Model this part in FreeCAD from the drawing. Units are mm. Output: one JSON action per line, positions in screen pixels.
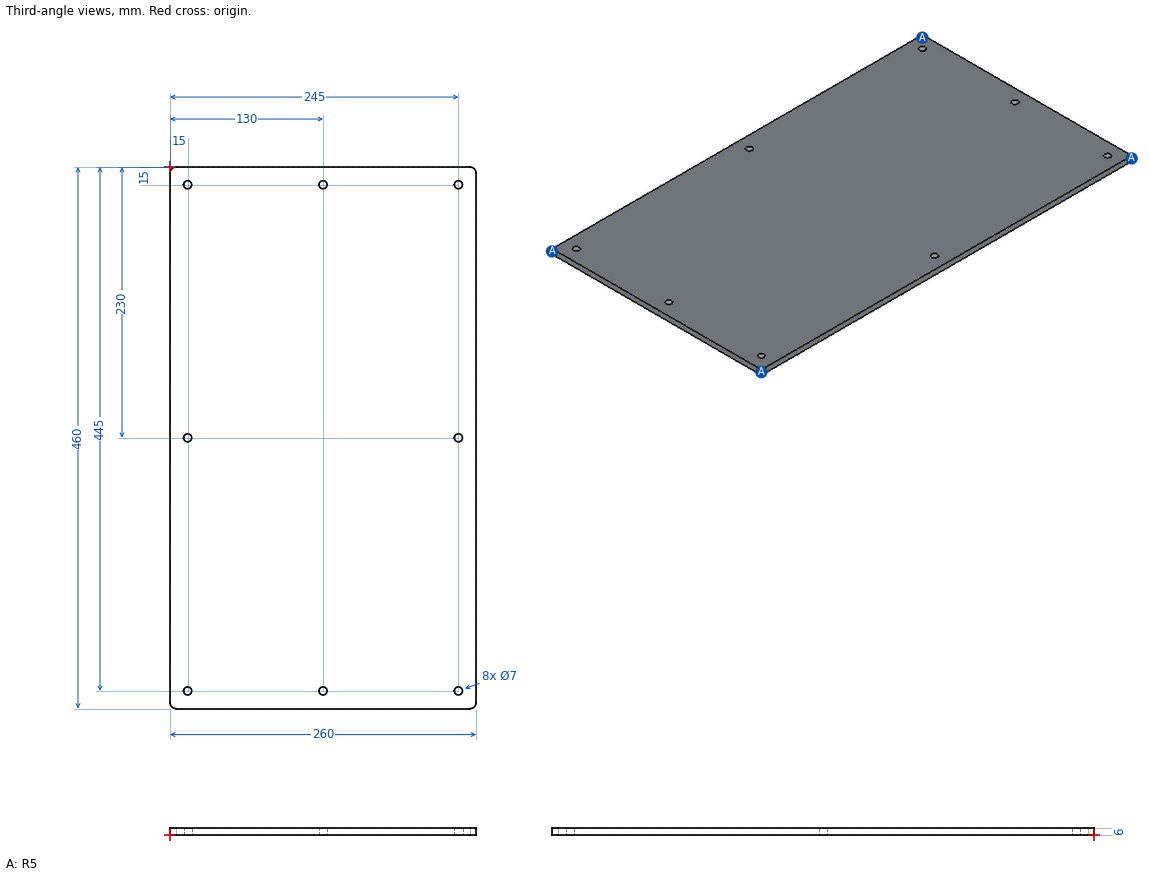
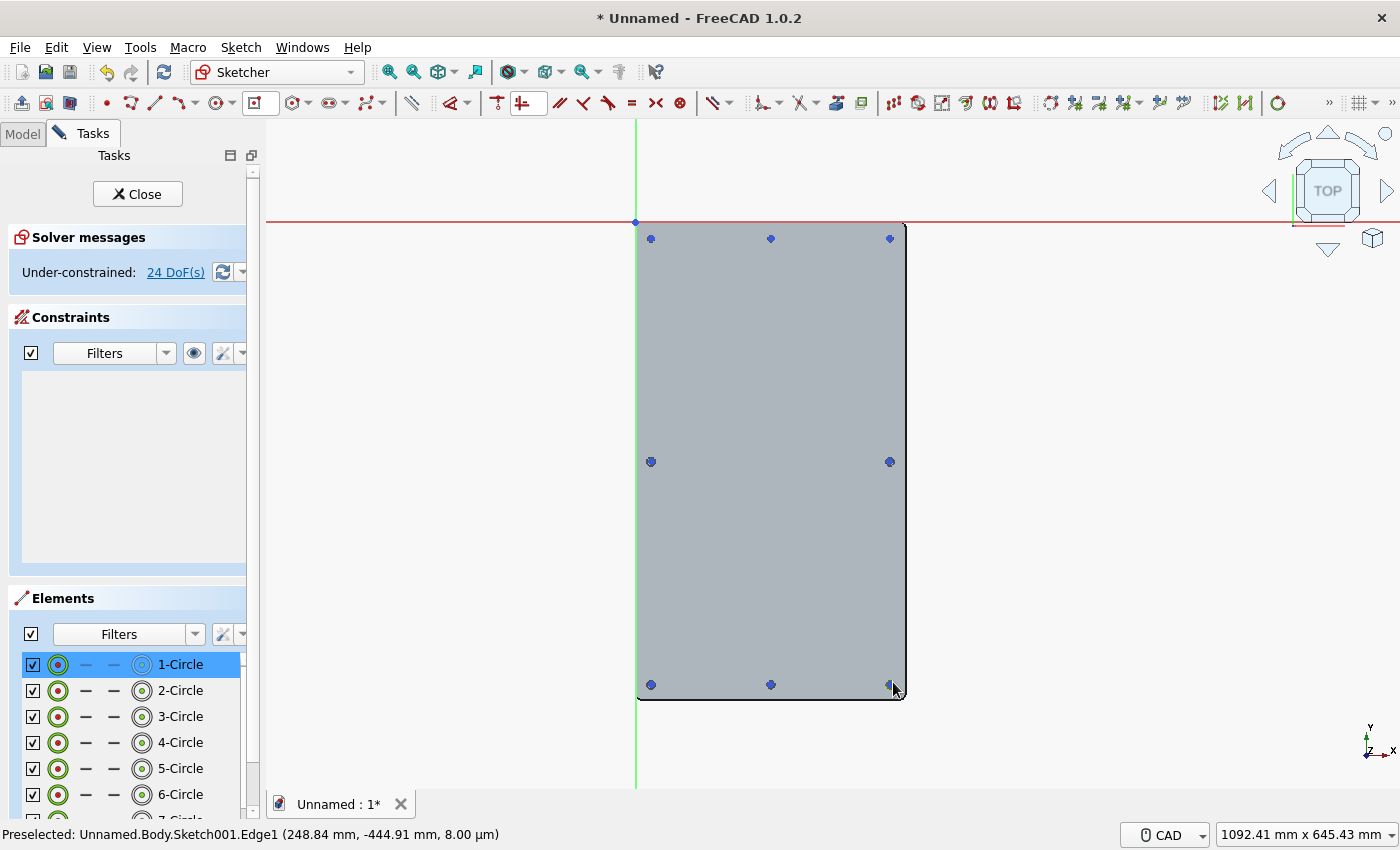
{"action": "scroll", "coordinate": [654, 682], "scroll_direction": "up", "scroll_amount": 7}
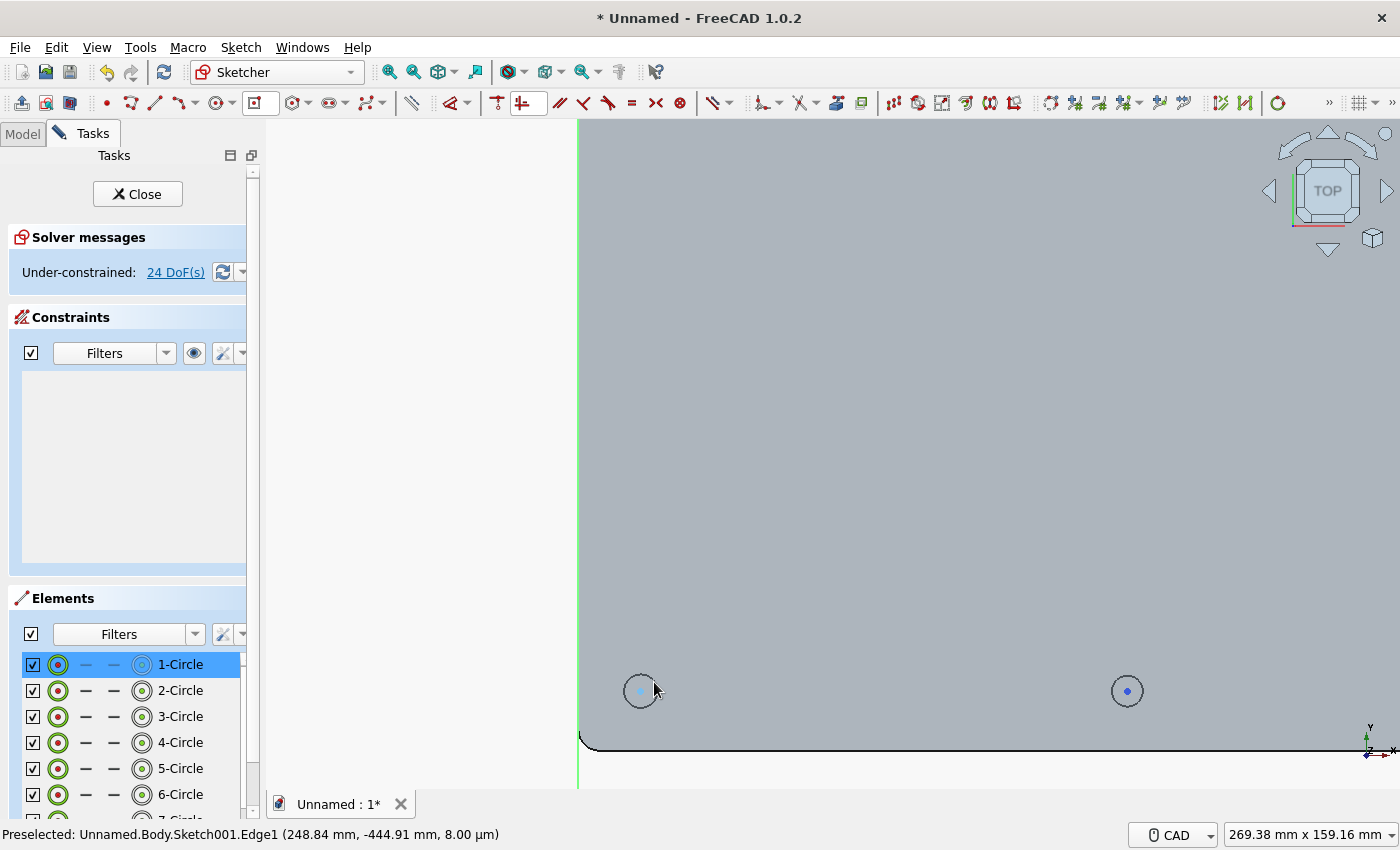
{"action": "left_click", "coordinate": [653, 679]}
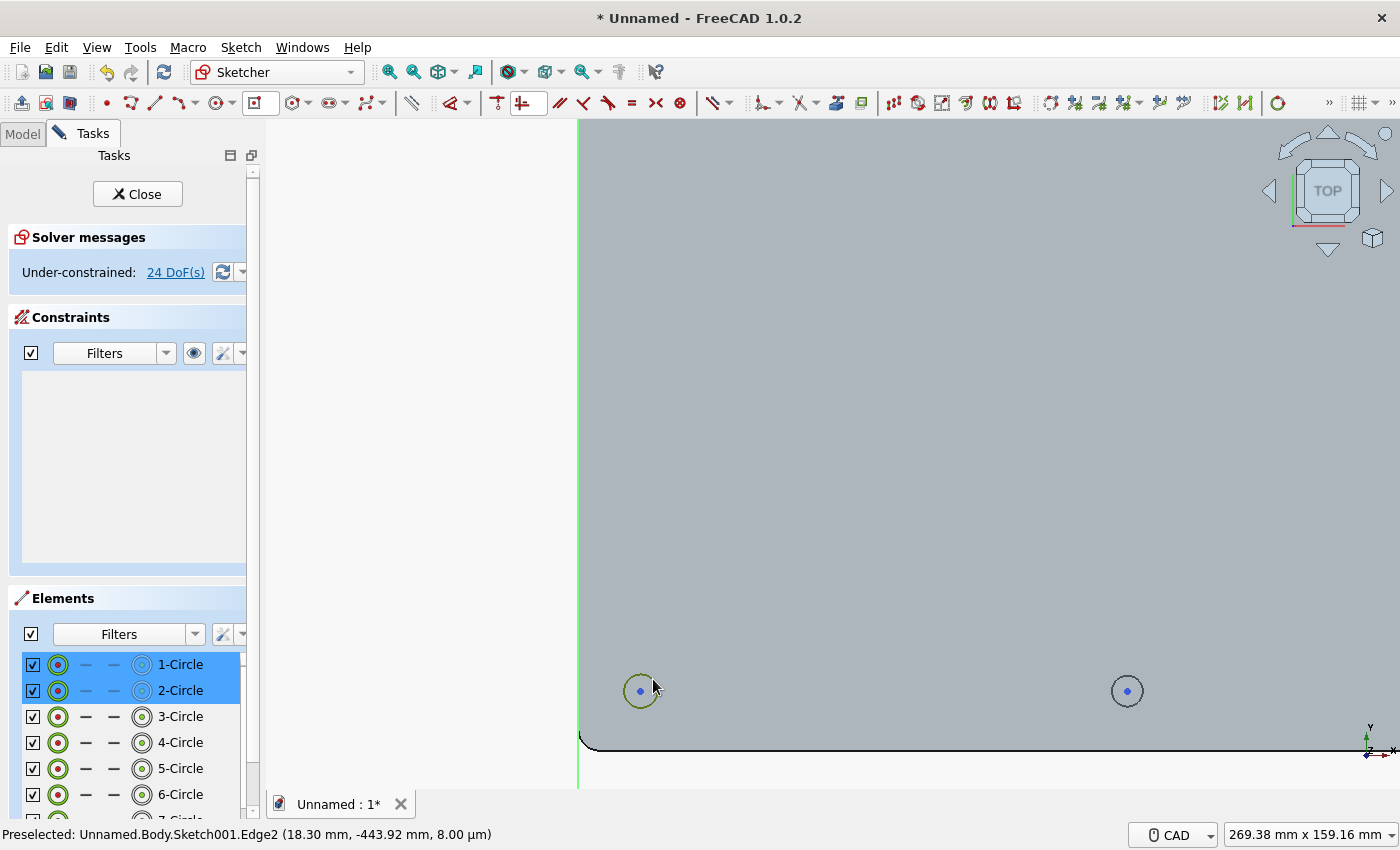
{"action": "scroll", "coordinate": [654, 682], "scroll_direction": "down", "scroll_amount": 7}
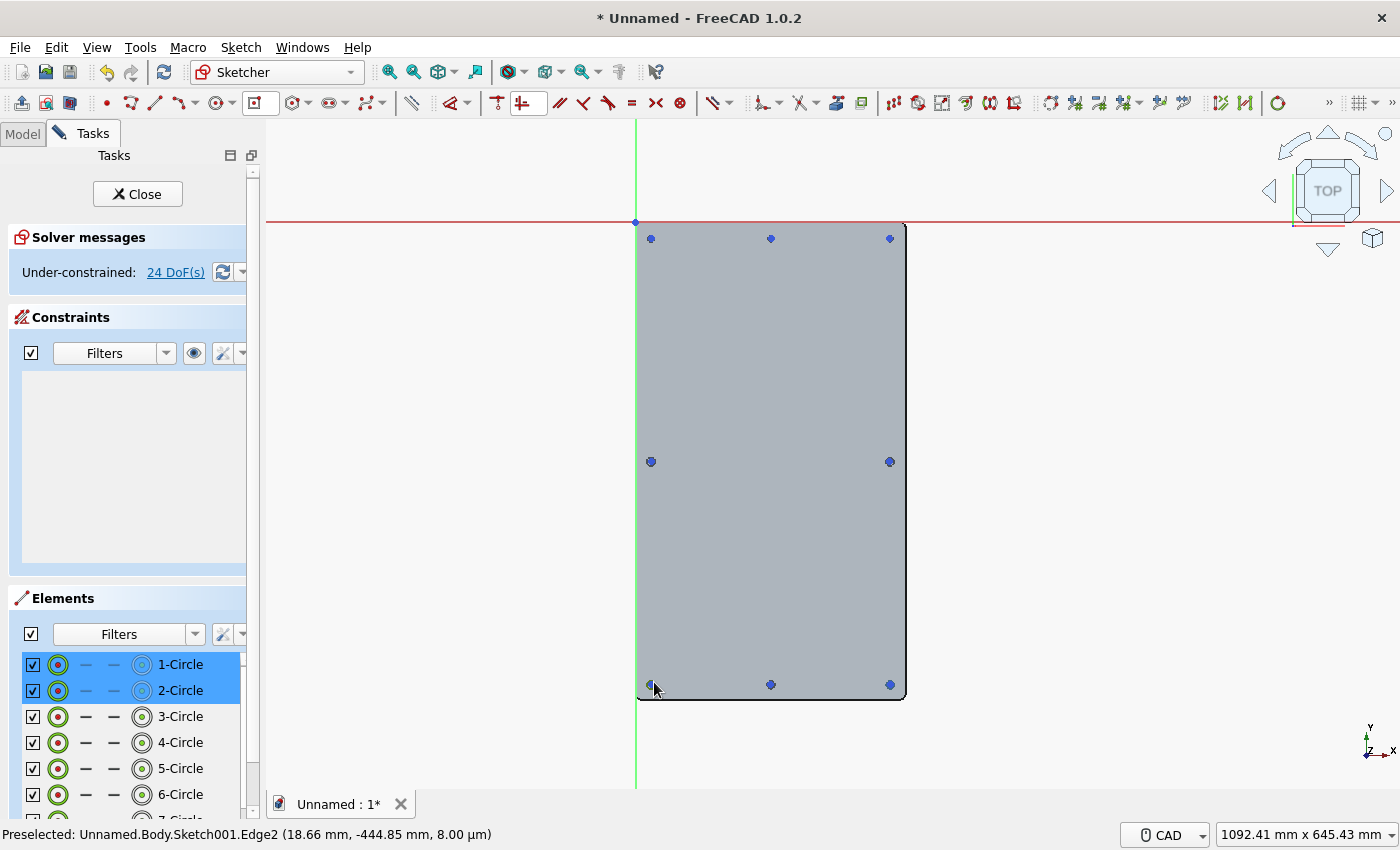
{"action": "scroll", "coordinate": [892, 237], "scroll_direction": "up", "scroll_amount": 8}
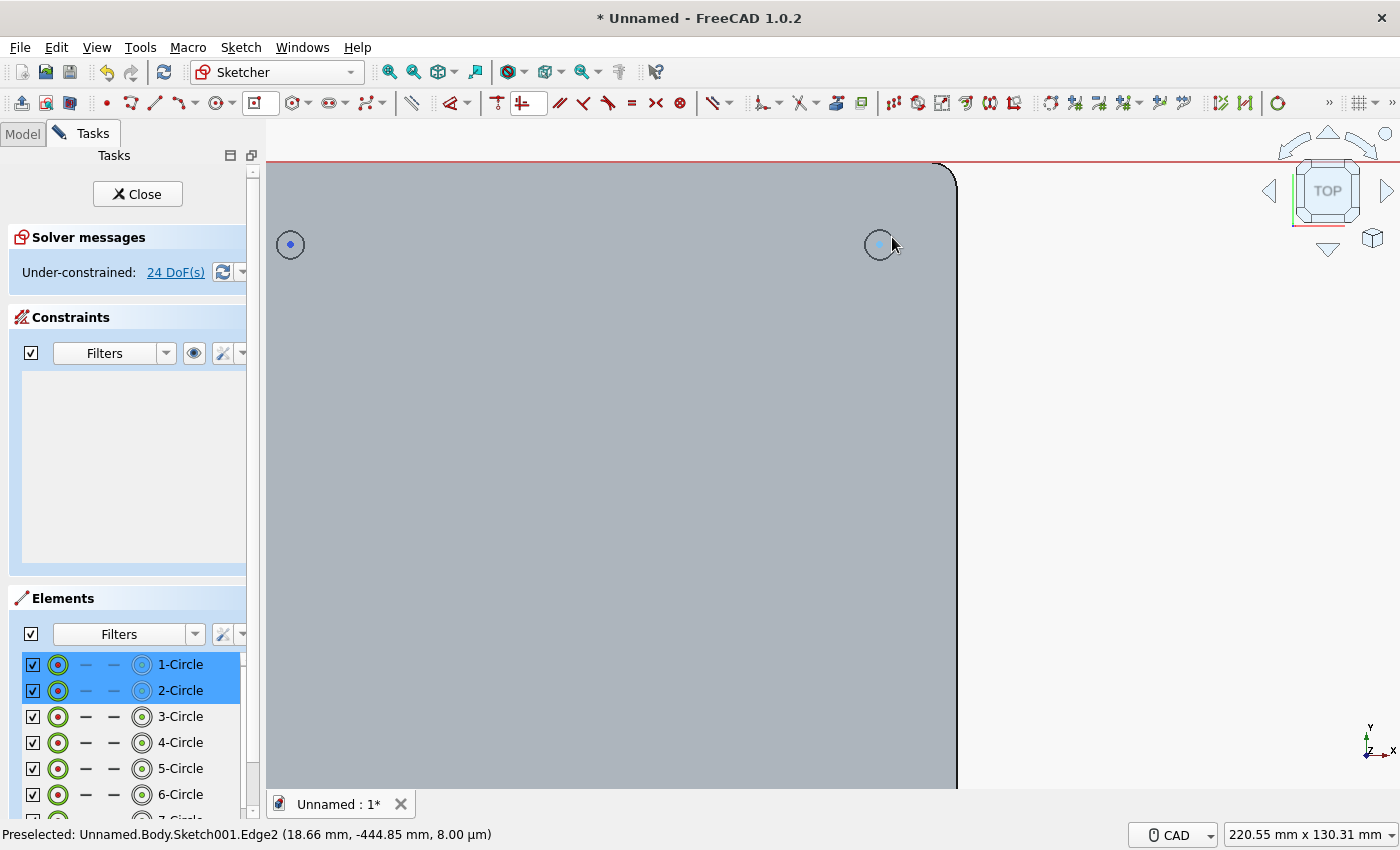
{"action": "left_click", "coordinate": [890, 234]}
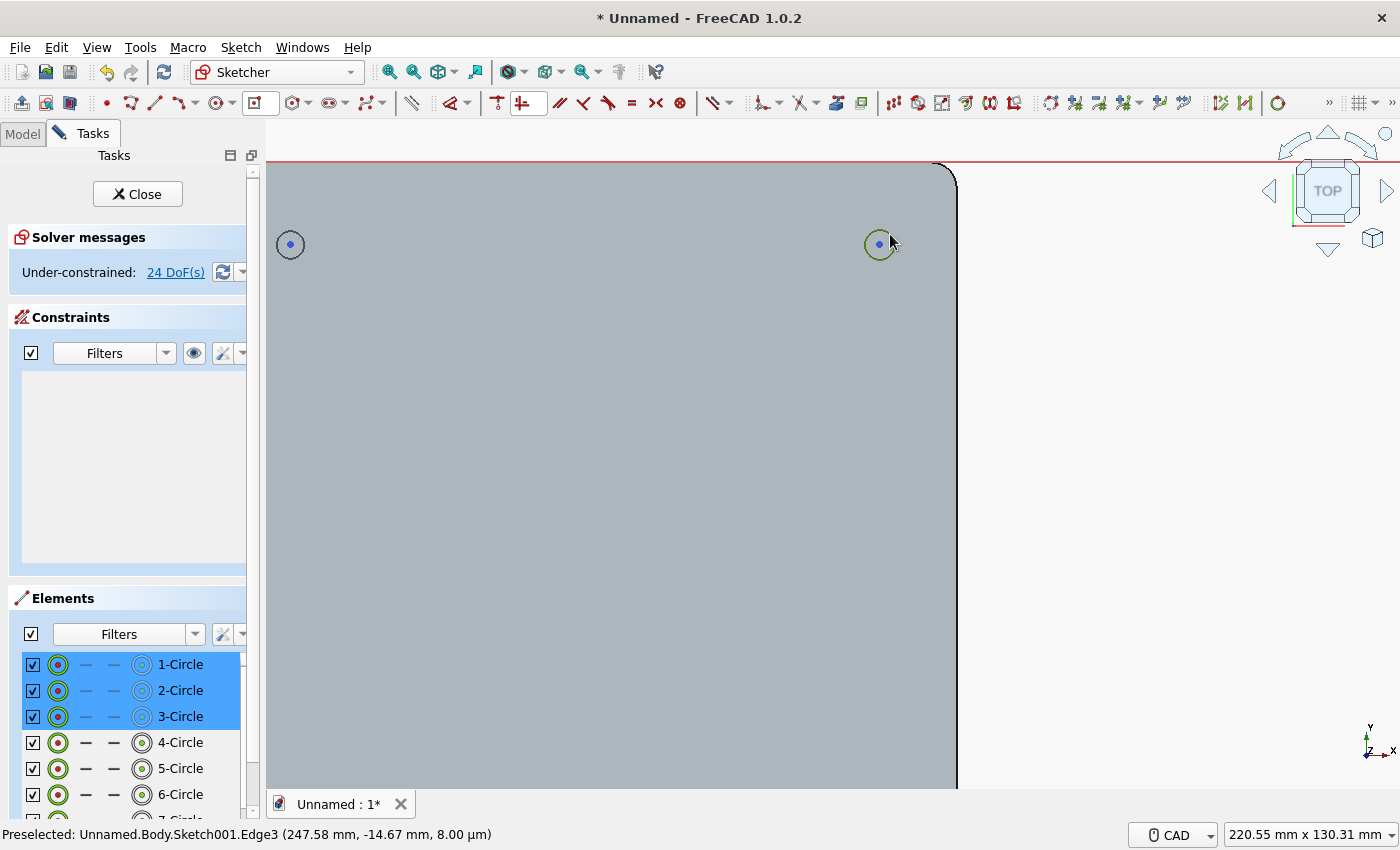
{"action": "scroll", "coordinate": [892, 236], "scroll_direction": "down", "scroll_amount": 8}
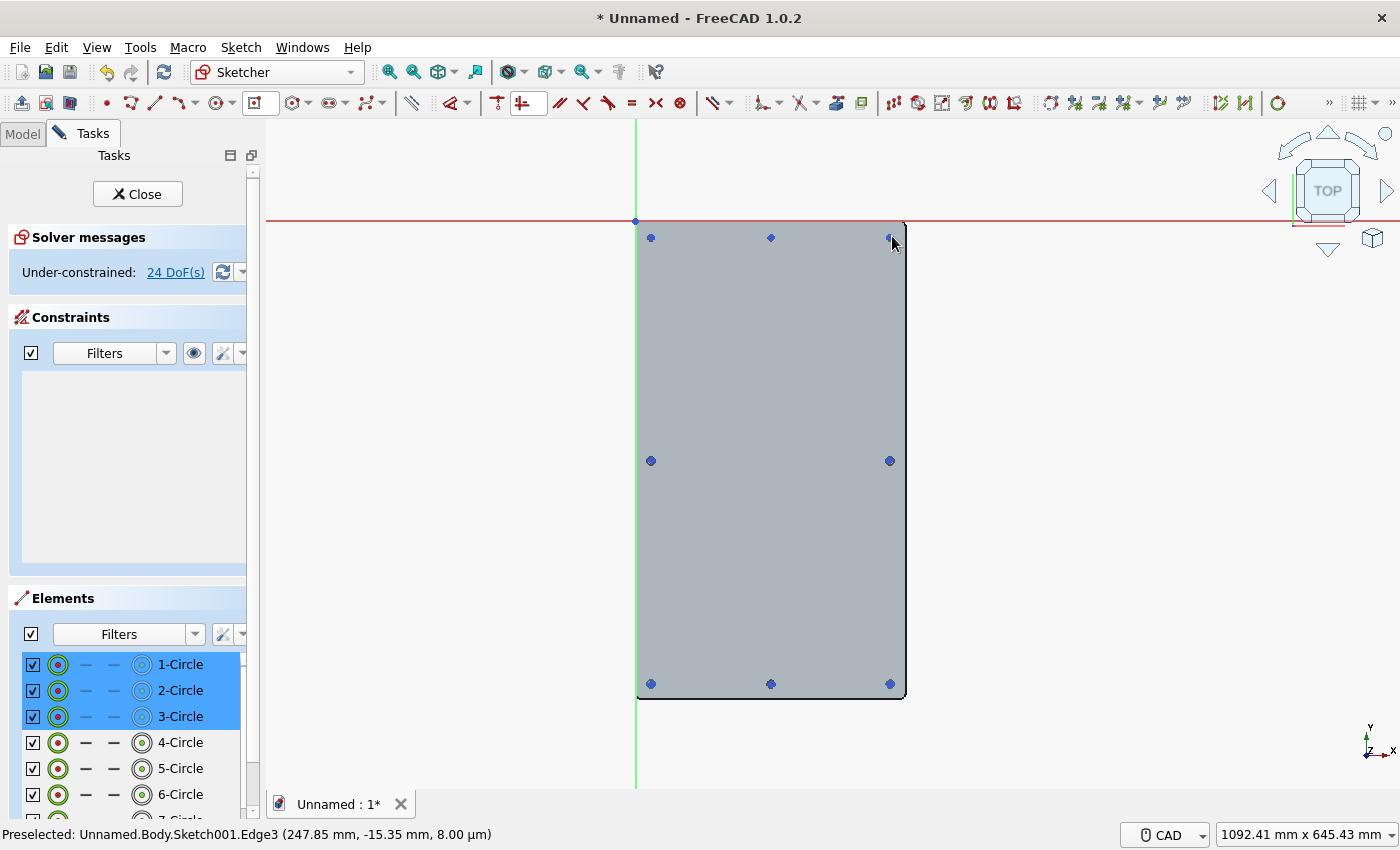
{"action": "scroll", "coordinate": [653, 236], "scroll_direction": "up", "scroll_amount": 8}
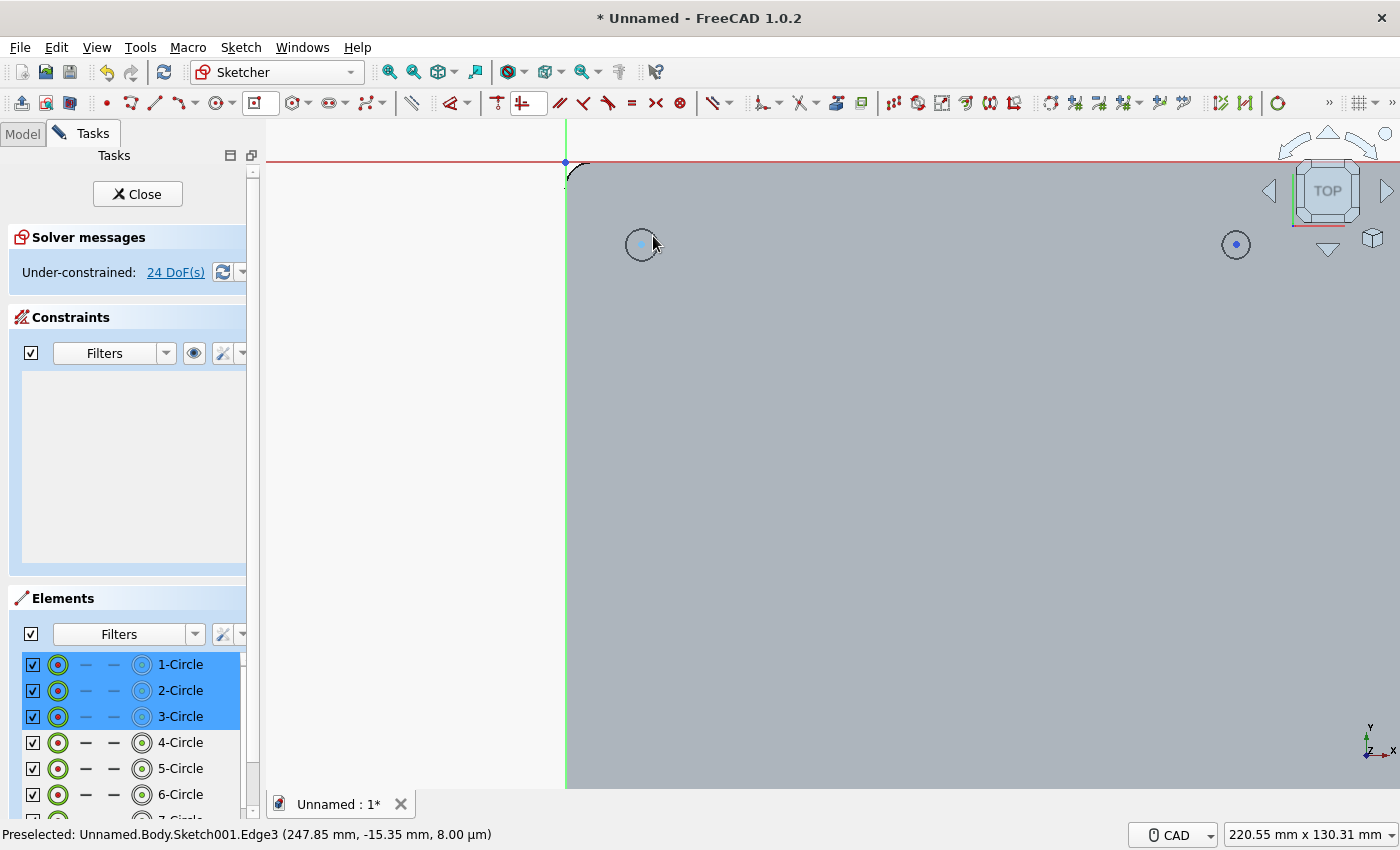
{"action": "left_click", "coordinate": [653, 234]}